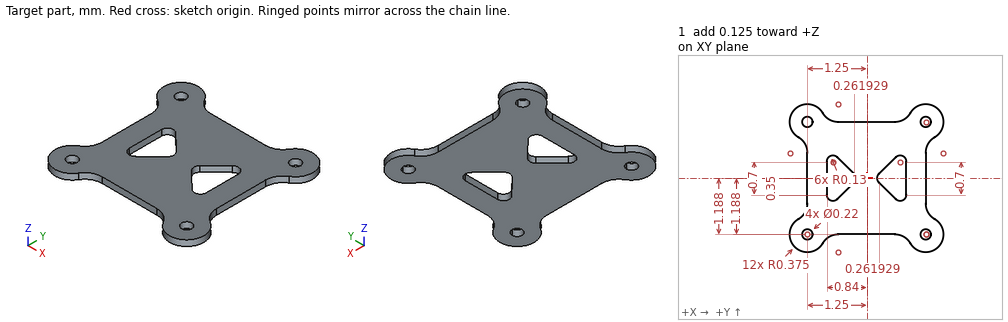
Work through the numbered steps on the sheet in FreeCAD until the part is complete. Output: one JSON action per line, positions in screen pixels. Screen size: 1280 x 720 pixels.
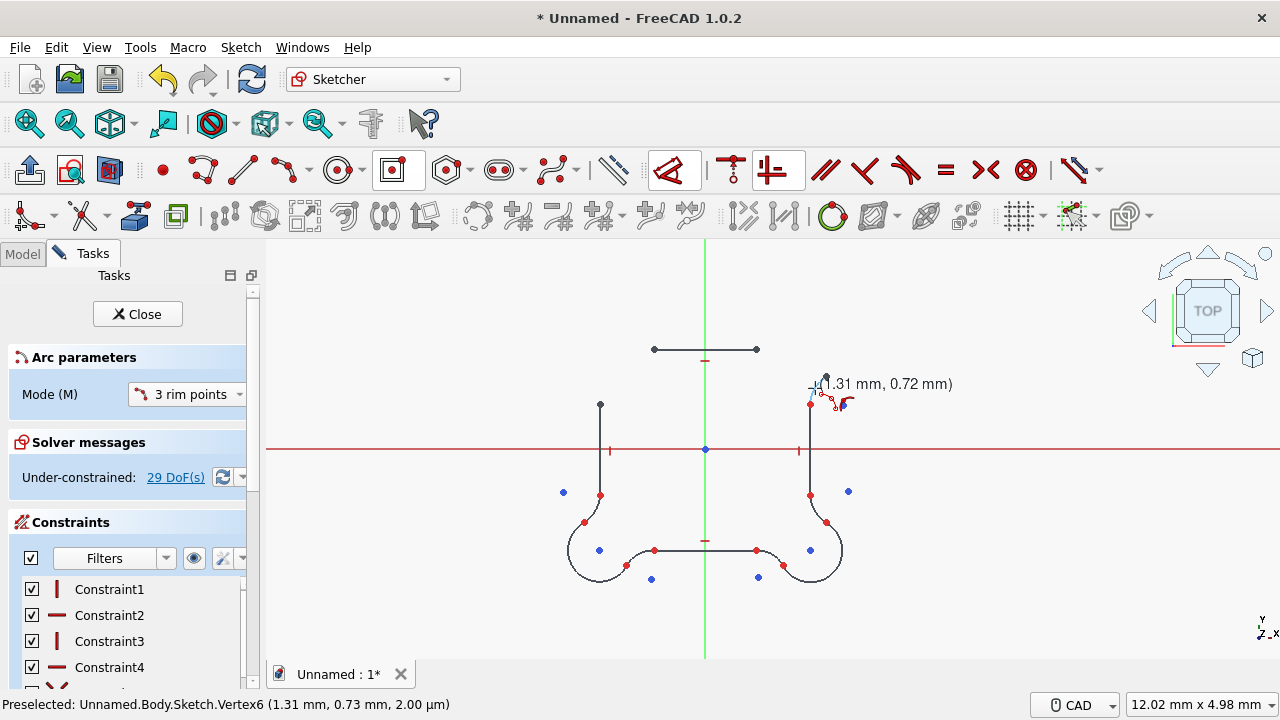
{"action": "left_click", "coordinate": [826, 377]}
{"action": "left_click", "coordinate": [783, 333]}
{"action": "left_click", "coordinate": [833, 327]}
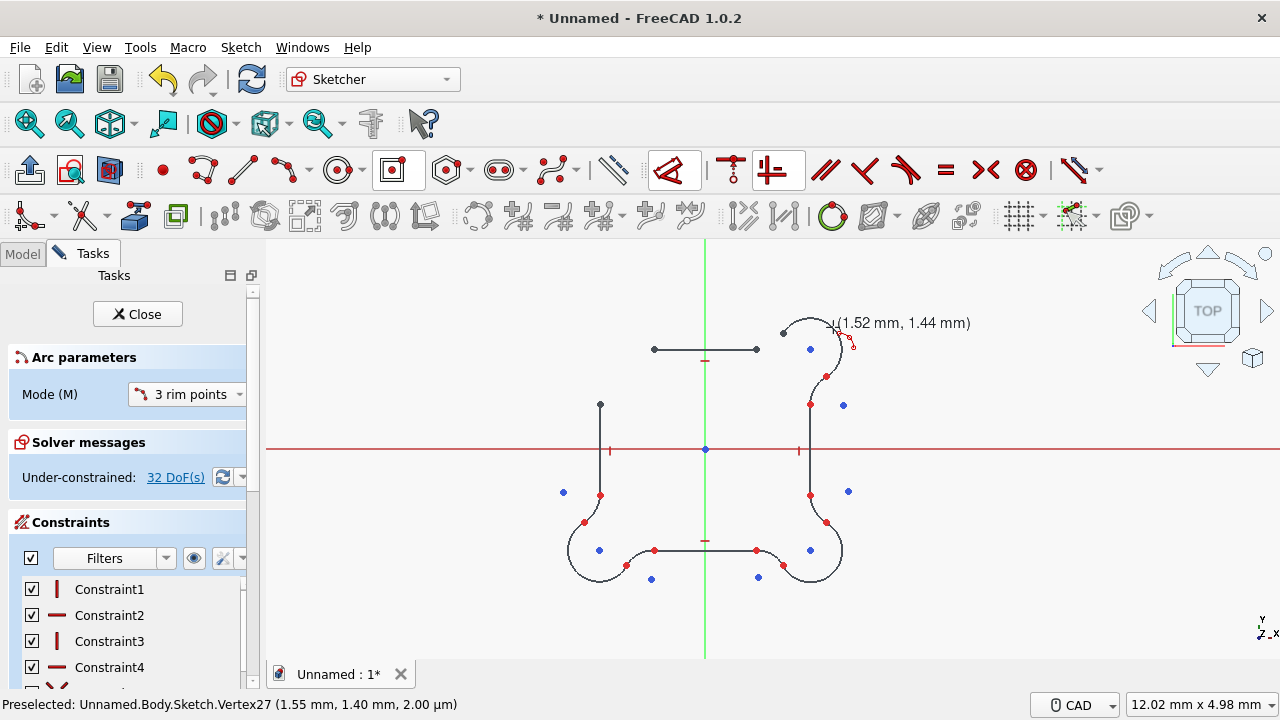
{"action": "left_click", "coordinate": [783, 334]}
{"action": "left_click", "coordinate": [756, 350]}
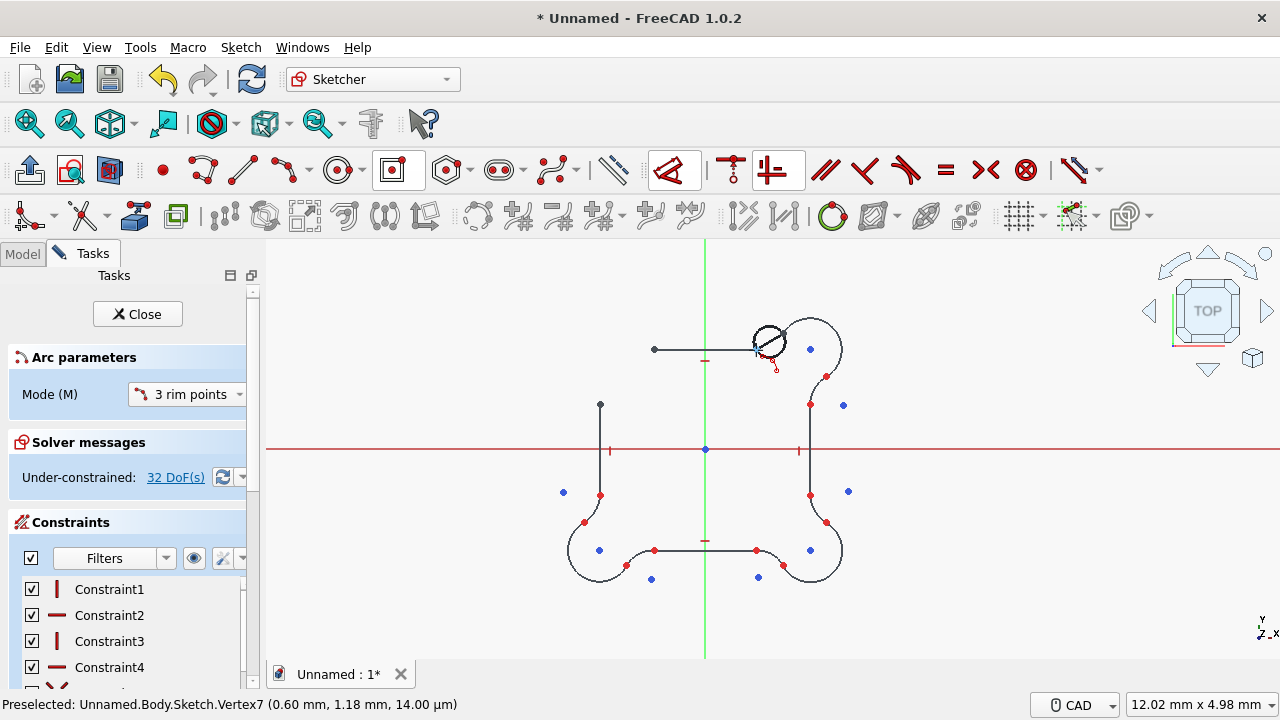
{"action": "scroll", "coordinate": [772, 345], "scroll_direction": "up", "scroll_amount": 7}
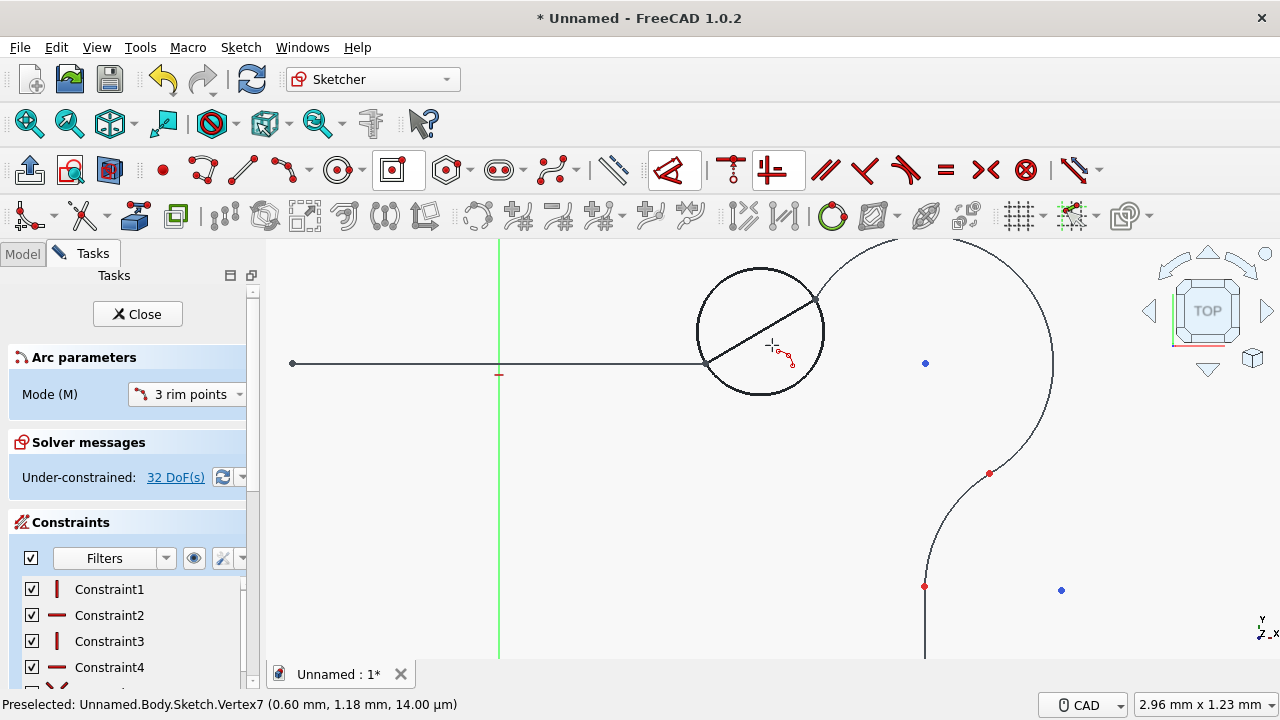
{"action": "left_click", "coordinate": [769, 343]}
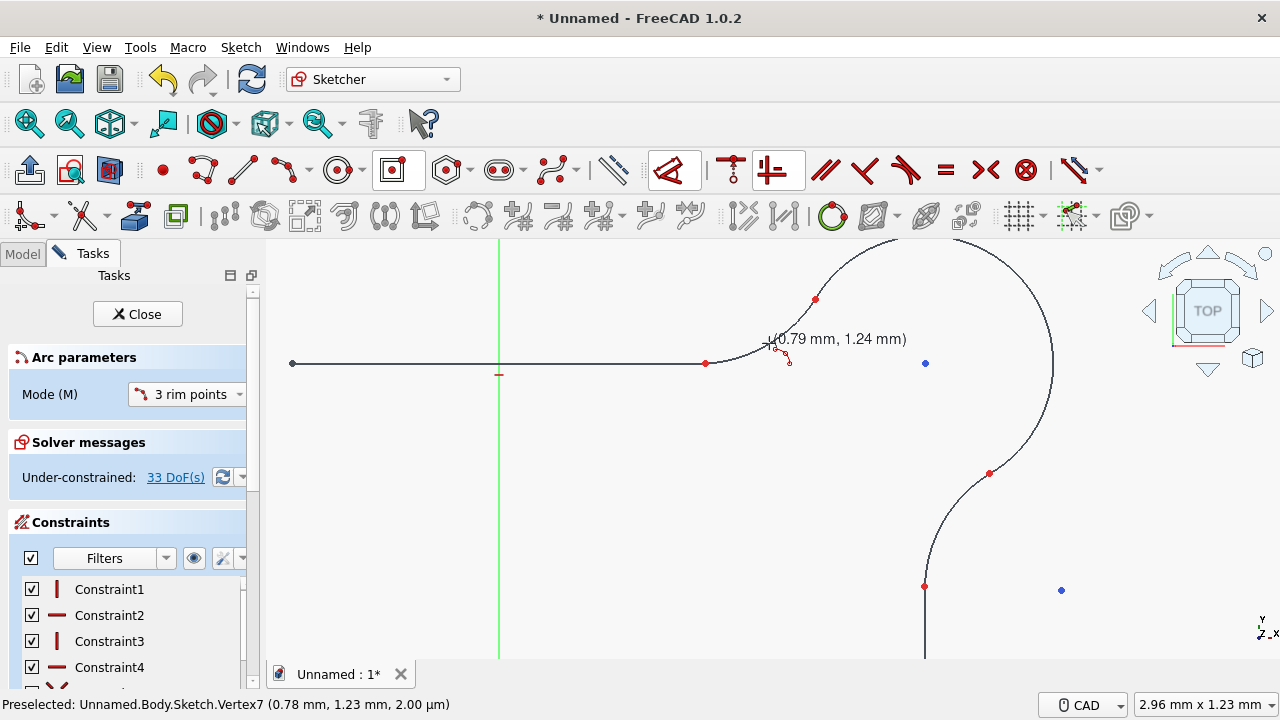
{"action": "scroll", "coordinate": [772, 345], "scroll_direction": "down", "scroll_amount": 7}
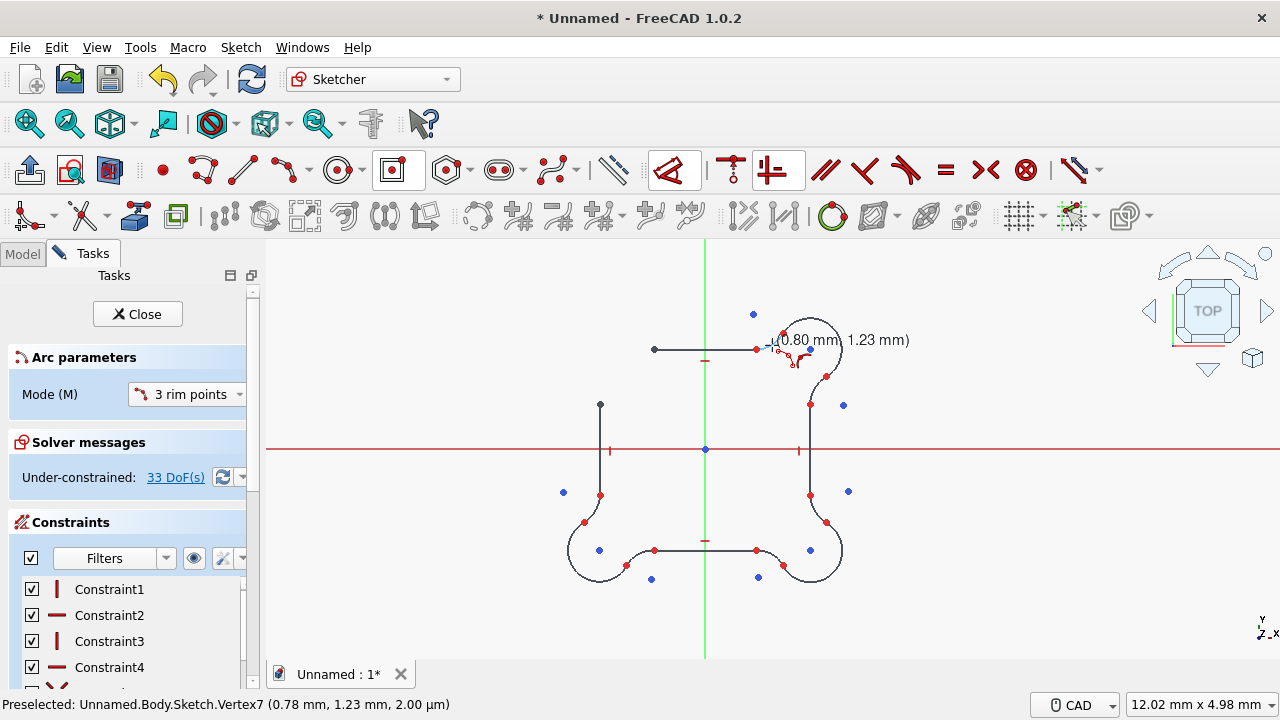
{"action": "left_click", "coordinate": [654, 350]}
{"action": "left_click", "coordinate": [627, 333]}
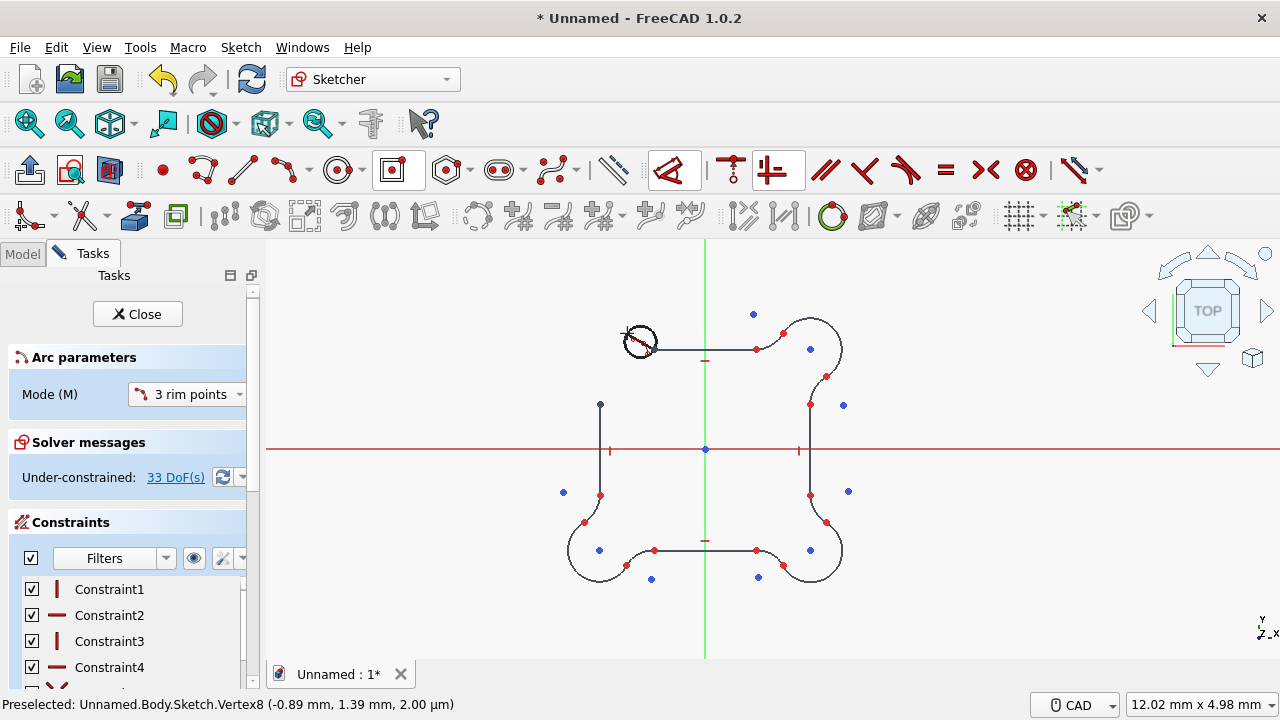
{"action": "scroll", "coordinate": [639, 345], "scroll_direction": "up", "scroll_amount": 7}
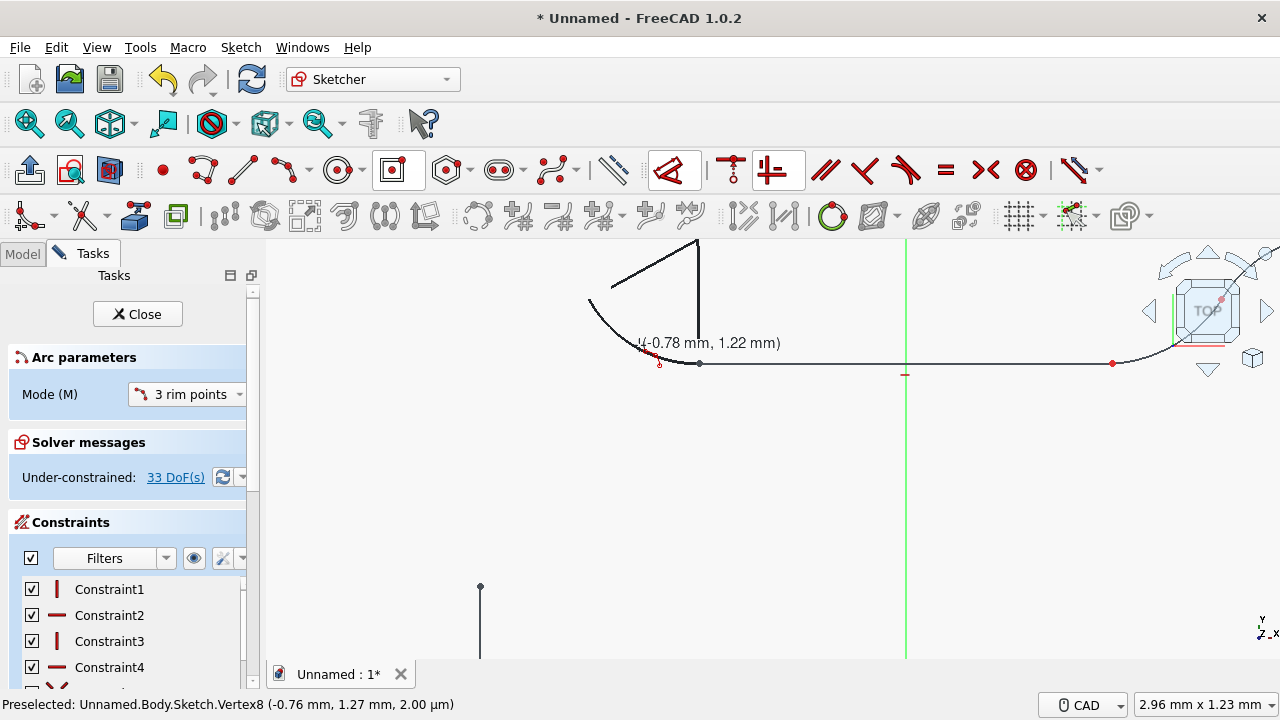
{"action": "left_click", "coordinate": [636, 343]}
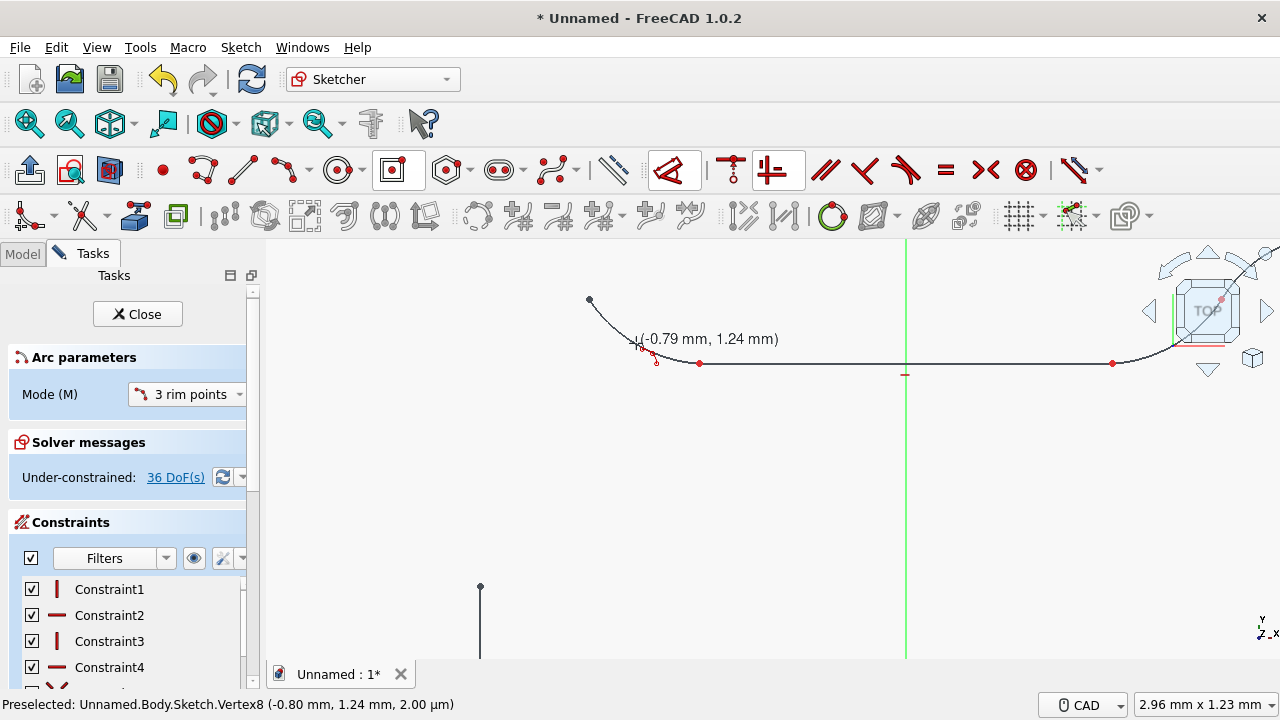
{"action": "scroll", "coordinate": [639, 345], "scroll_direction": "down", "scroll_amount": 7}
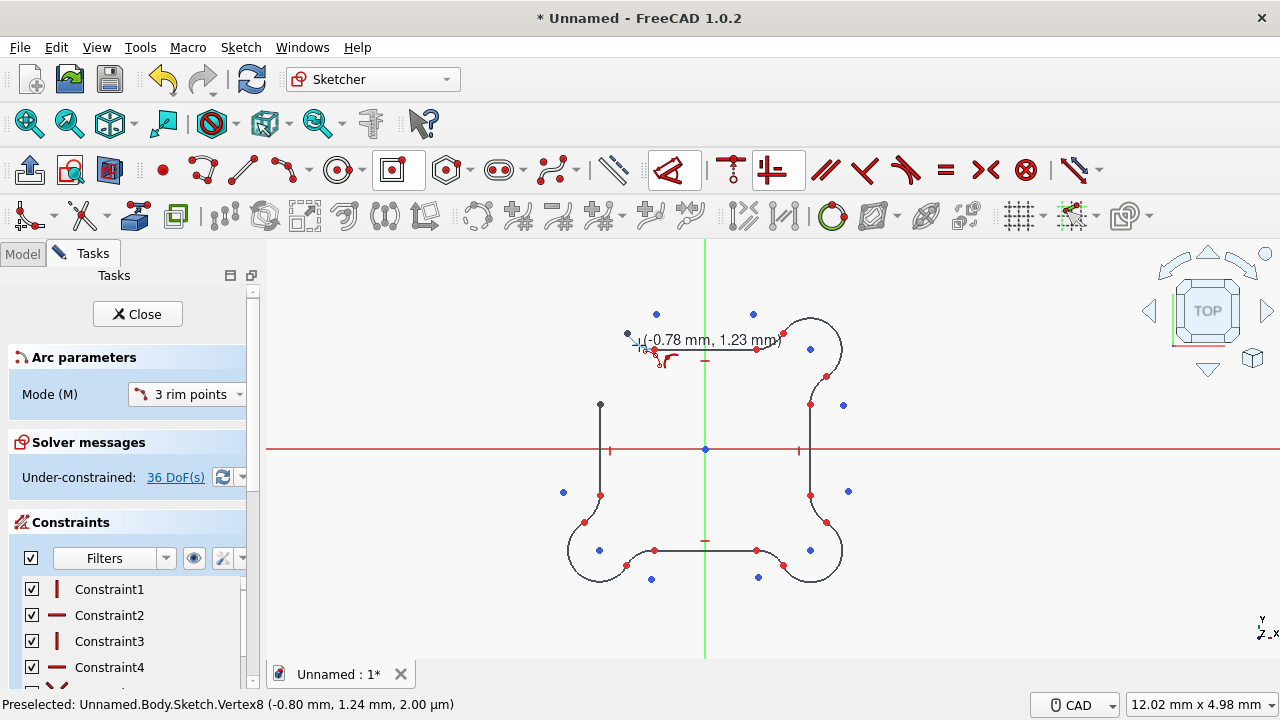
{"action": "left_click", "coordinate": [627, 334]}
{"action": "left_click", "coordinate": [584, 376]}
{"action": "left_click", "coordinate": [577, 327]}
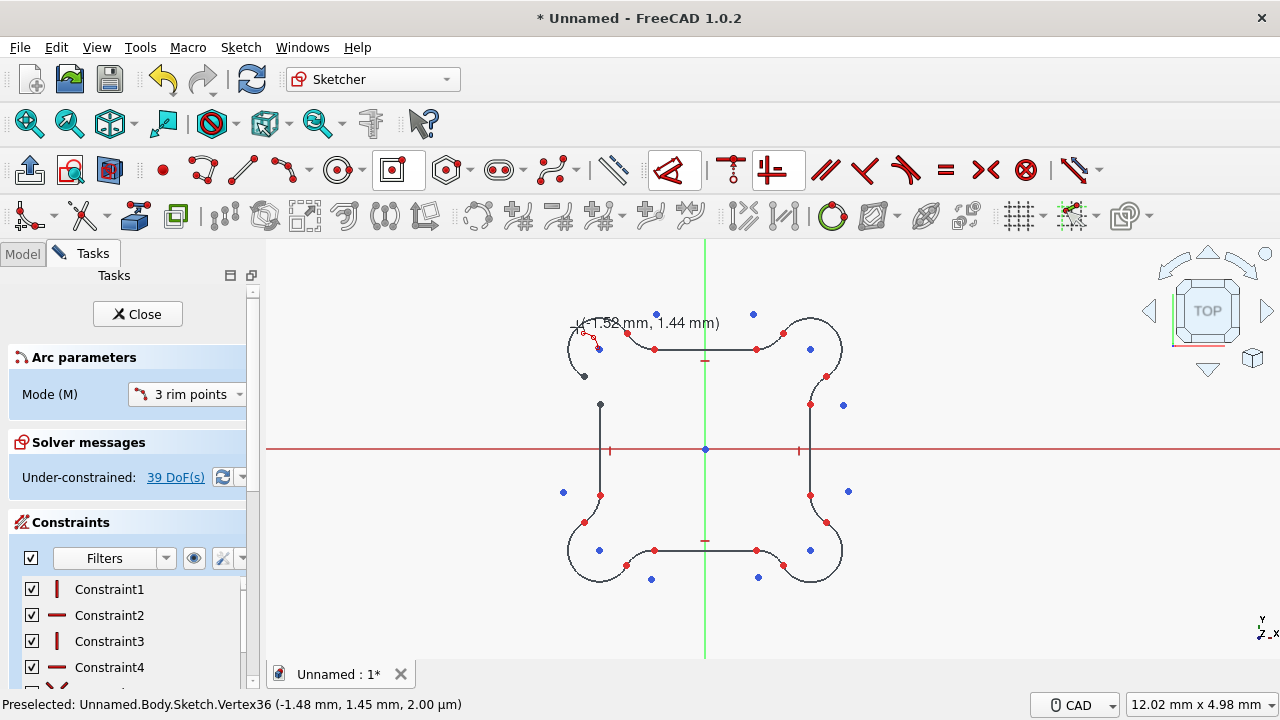
{"action": "left_click", "coordinate": [584, 377]}
{"action": "left_click", "coordinate": [600, 405]}